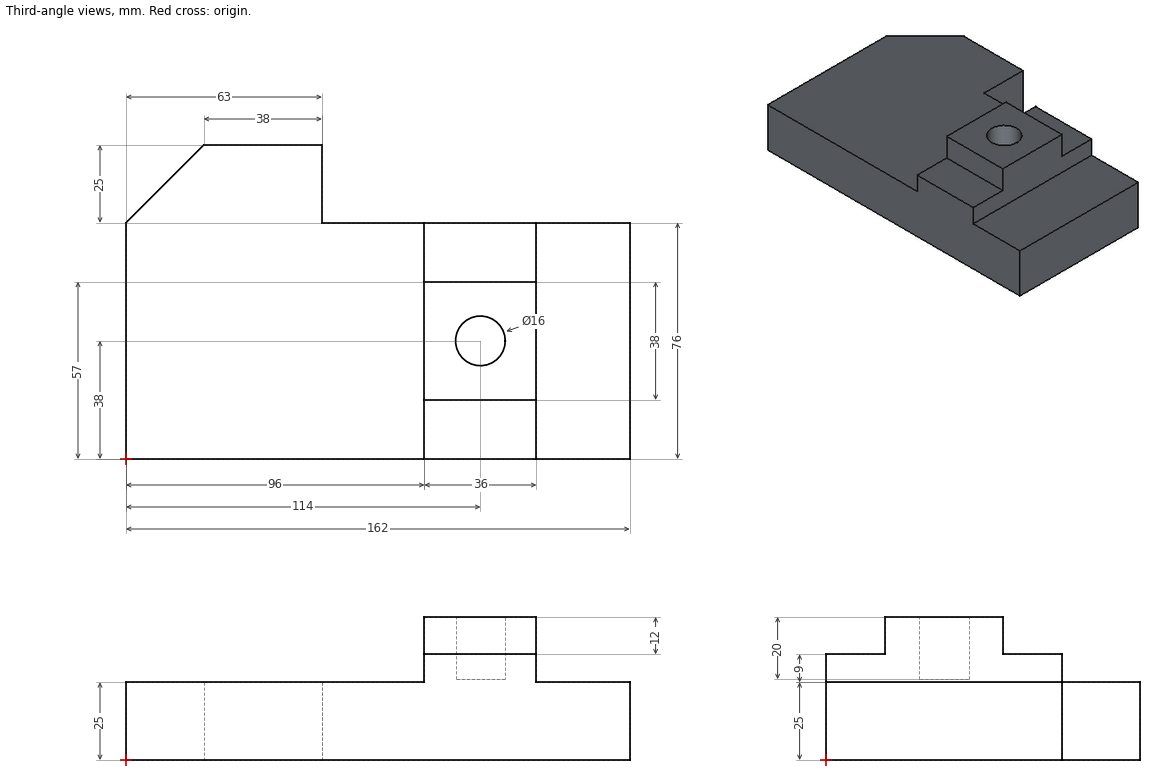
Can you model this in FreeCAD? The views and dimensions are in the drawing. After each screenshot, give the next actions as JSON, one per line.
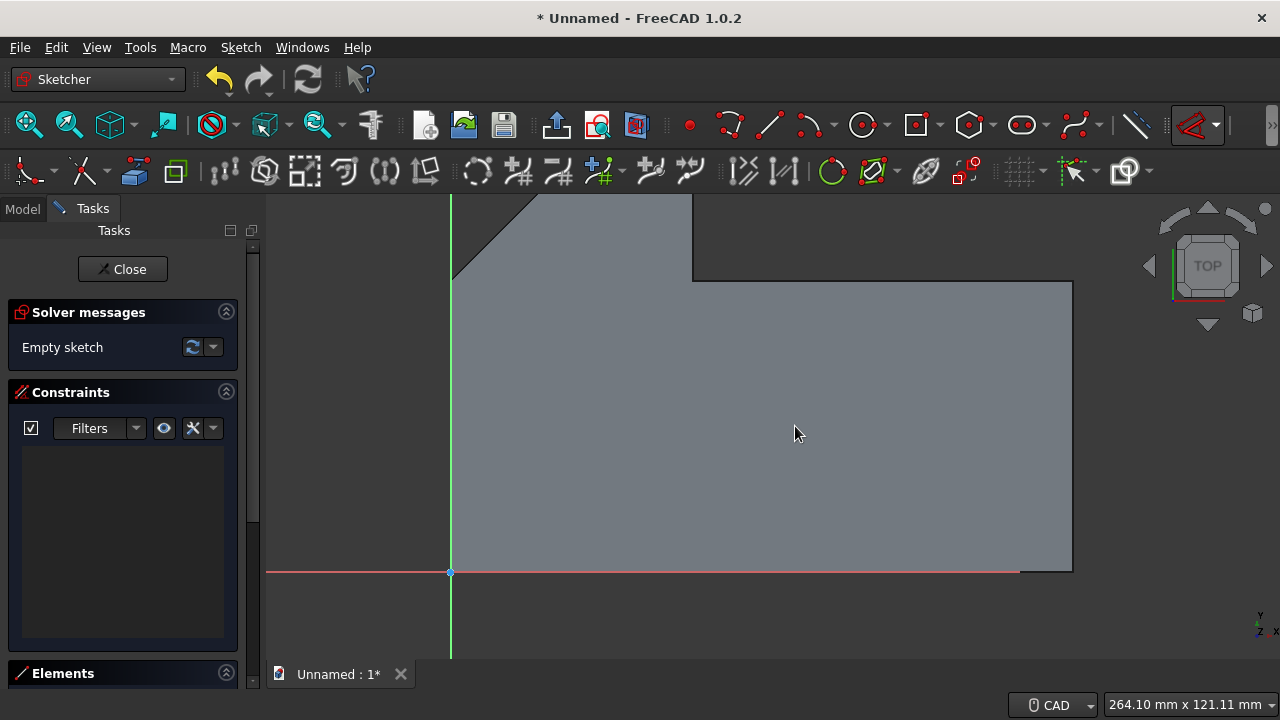
{"action": "key", "text": "g r"}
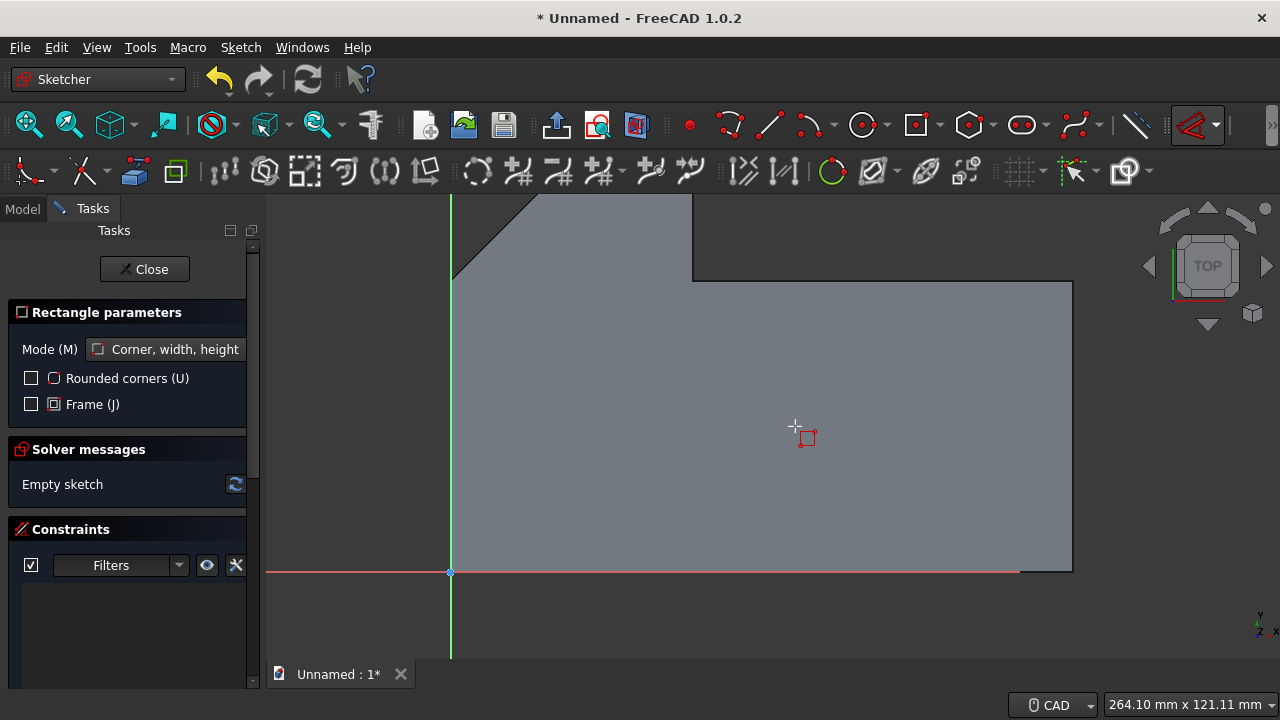
{"action": "left_click", "coordinate": [820, 281]}
{"action": "left_click", "coordinate": [958, 572]}
{"action": "key", "text": "Escape"}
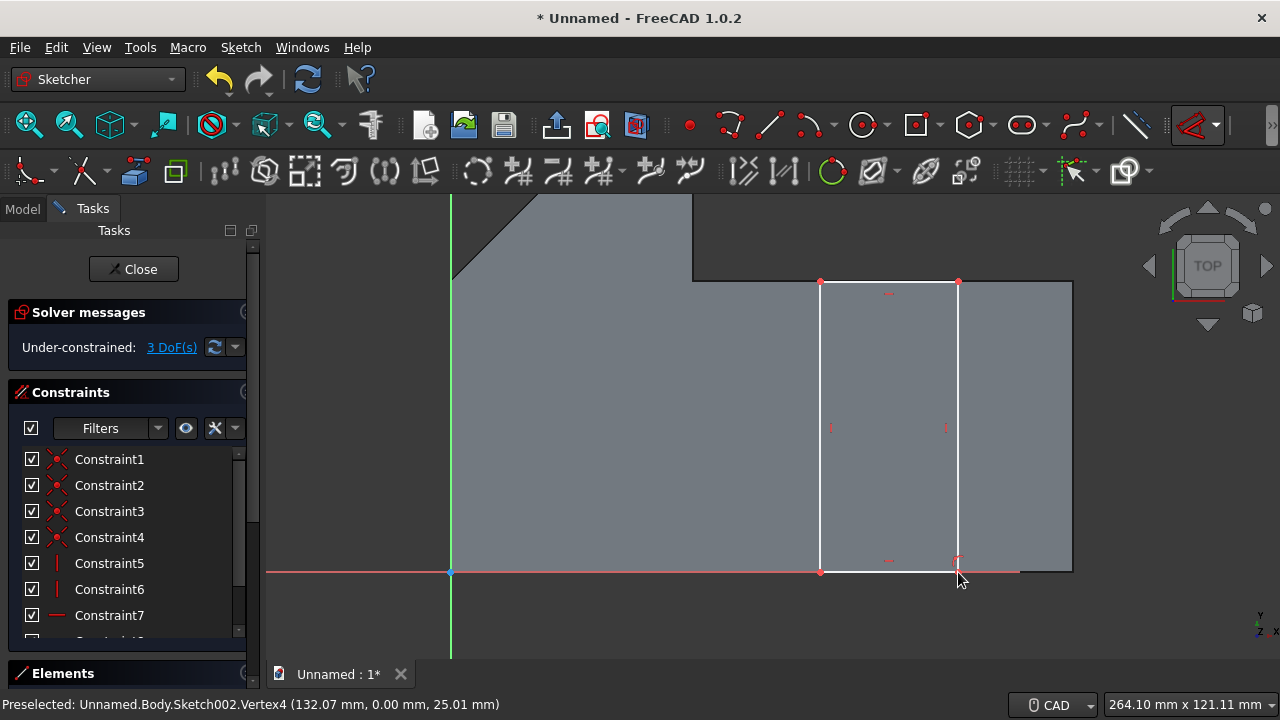
{"action": "left_click", "coordinate": [820, 369]}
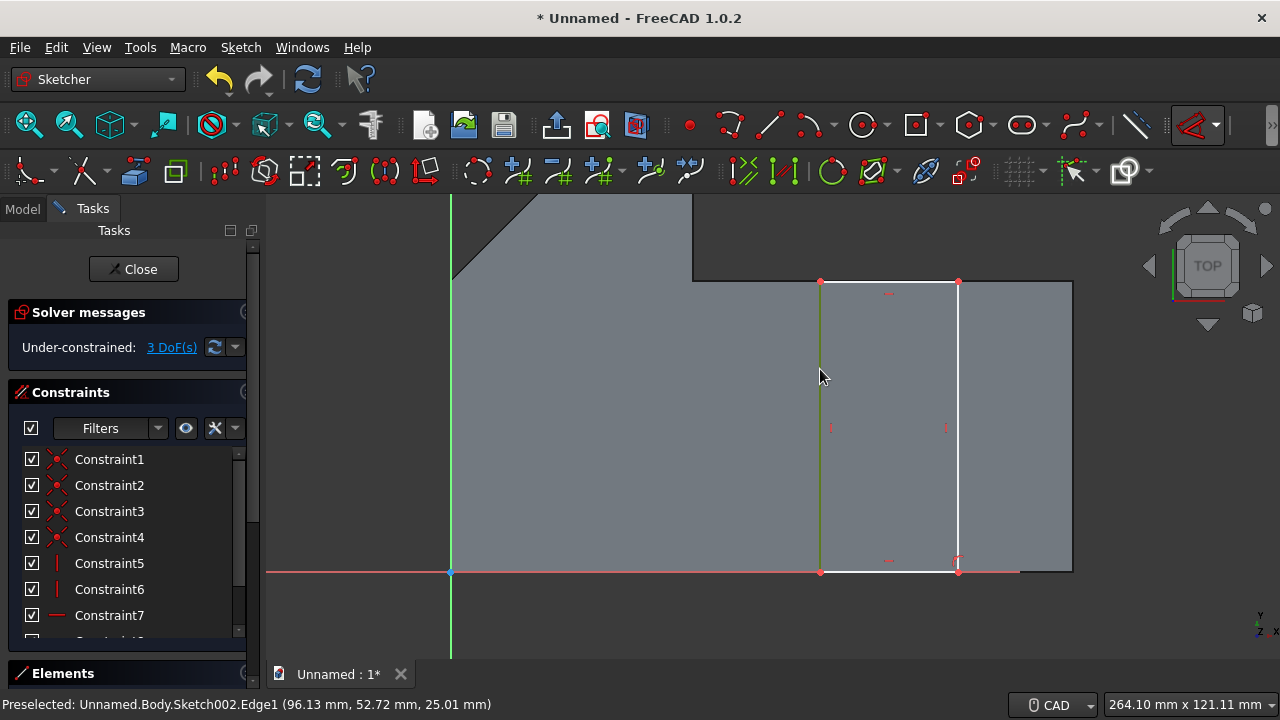
{"action": "left_click", "coordinate": [1218, 126]}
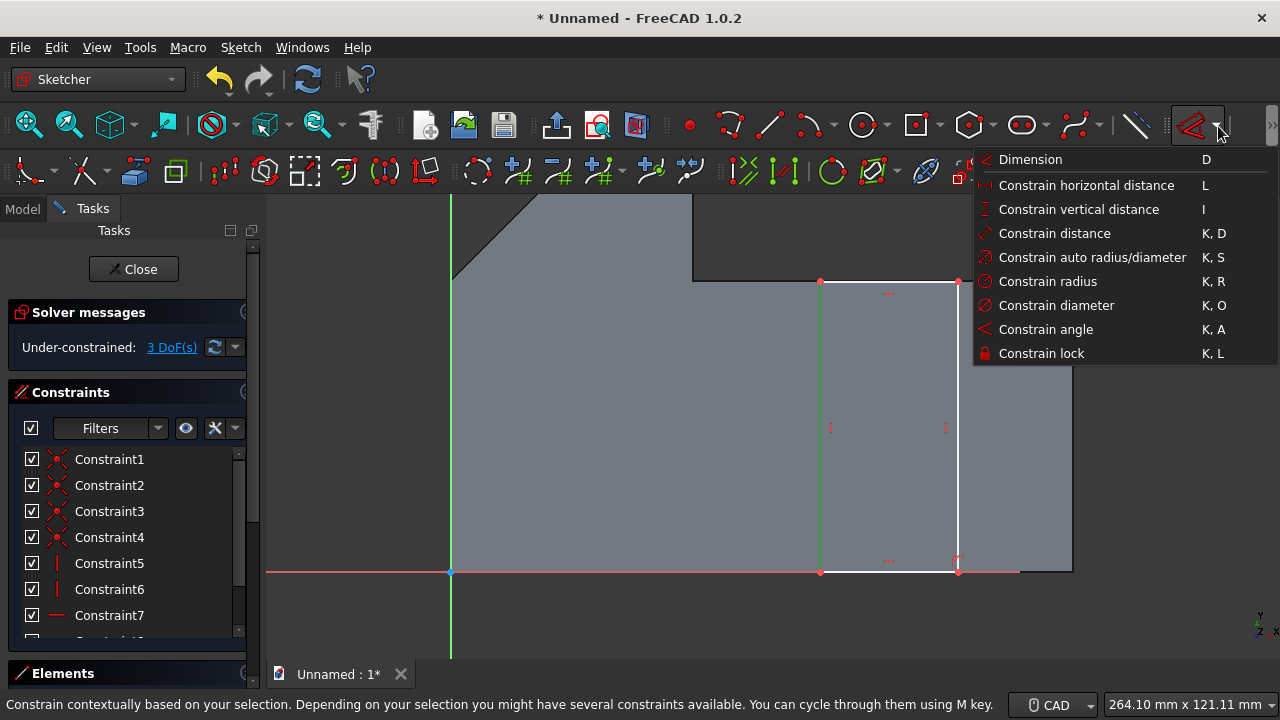
{"action": "left_click", "coordinate": [1126, 209]}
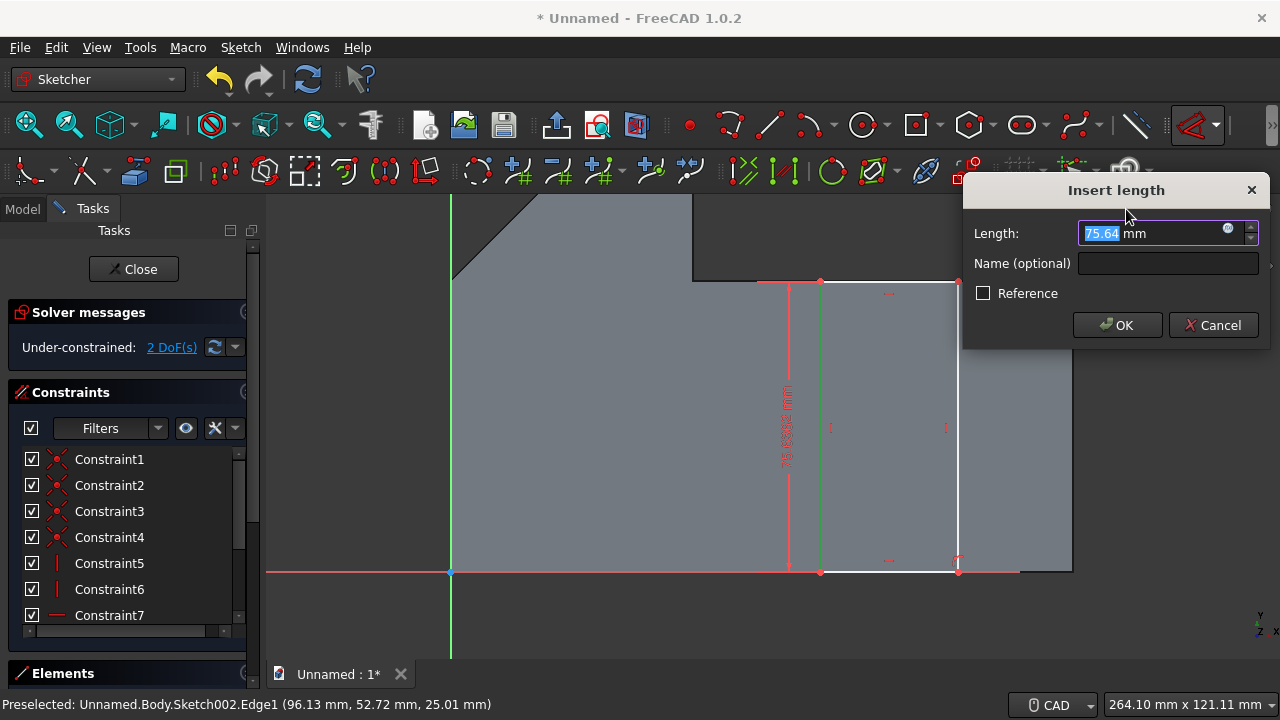
{"action": "type", "text": "76"}
{"action": "key", "text": "Return"}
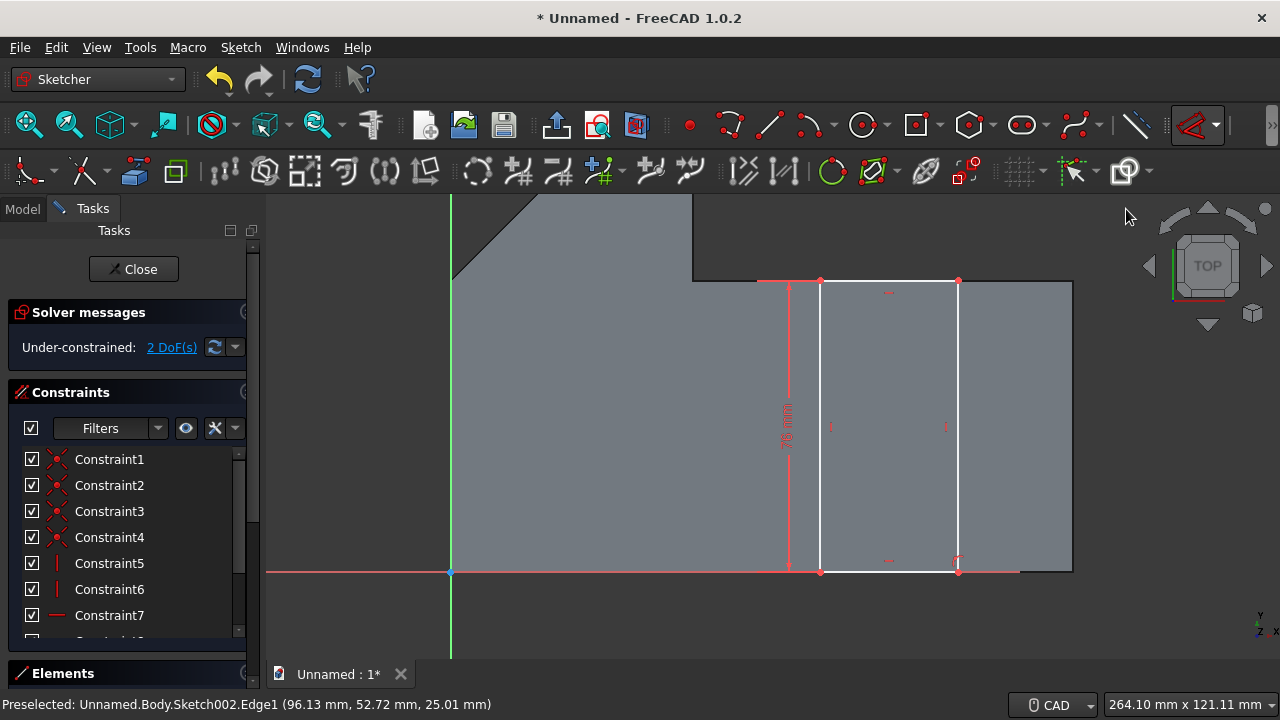
{"action": "left_click", "coordinate": [861, 572]}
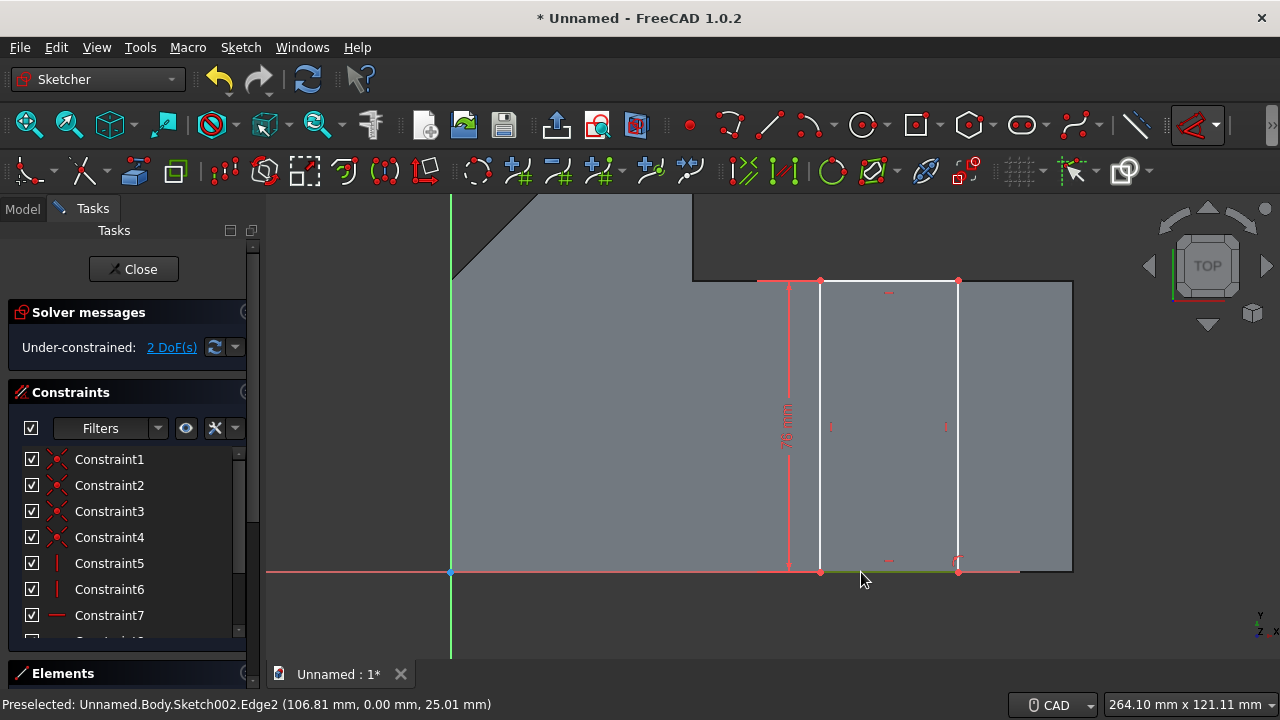
{"action": "key", "text": "l"}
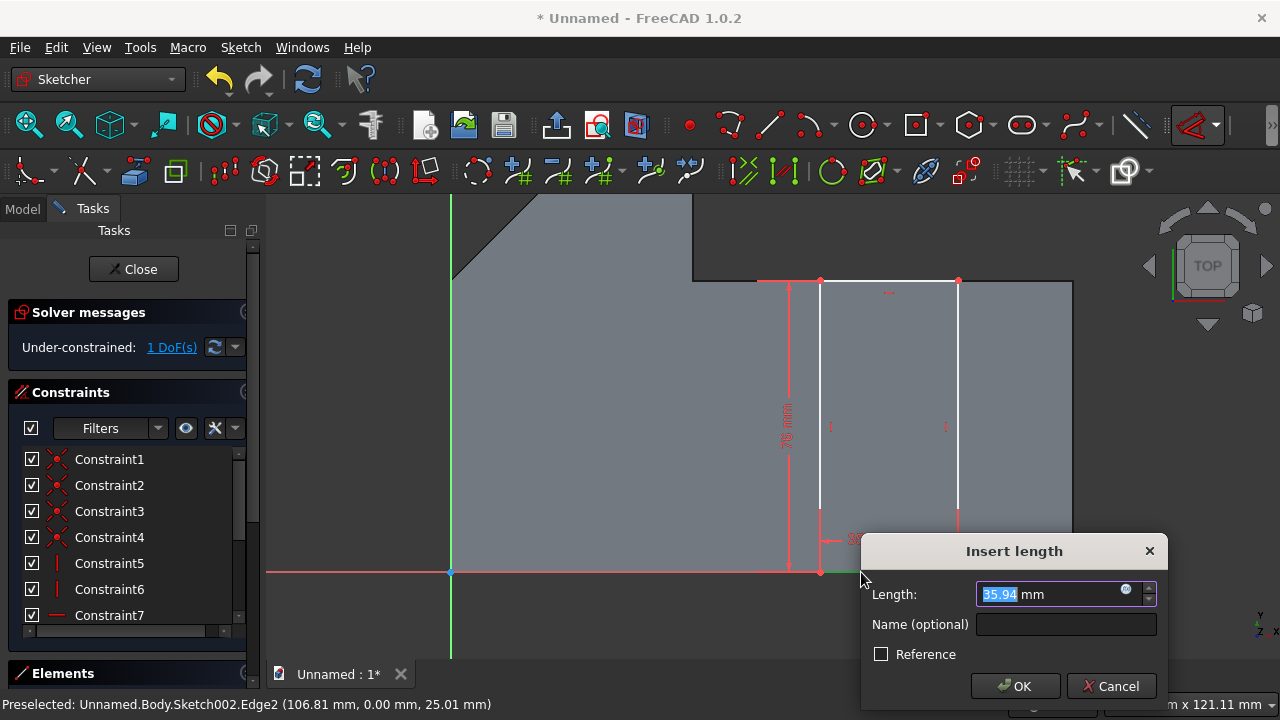
{"action": "type", "text": "36"}
{"action": "key", "text": "Return"}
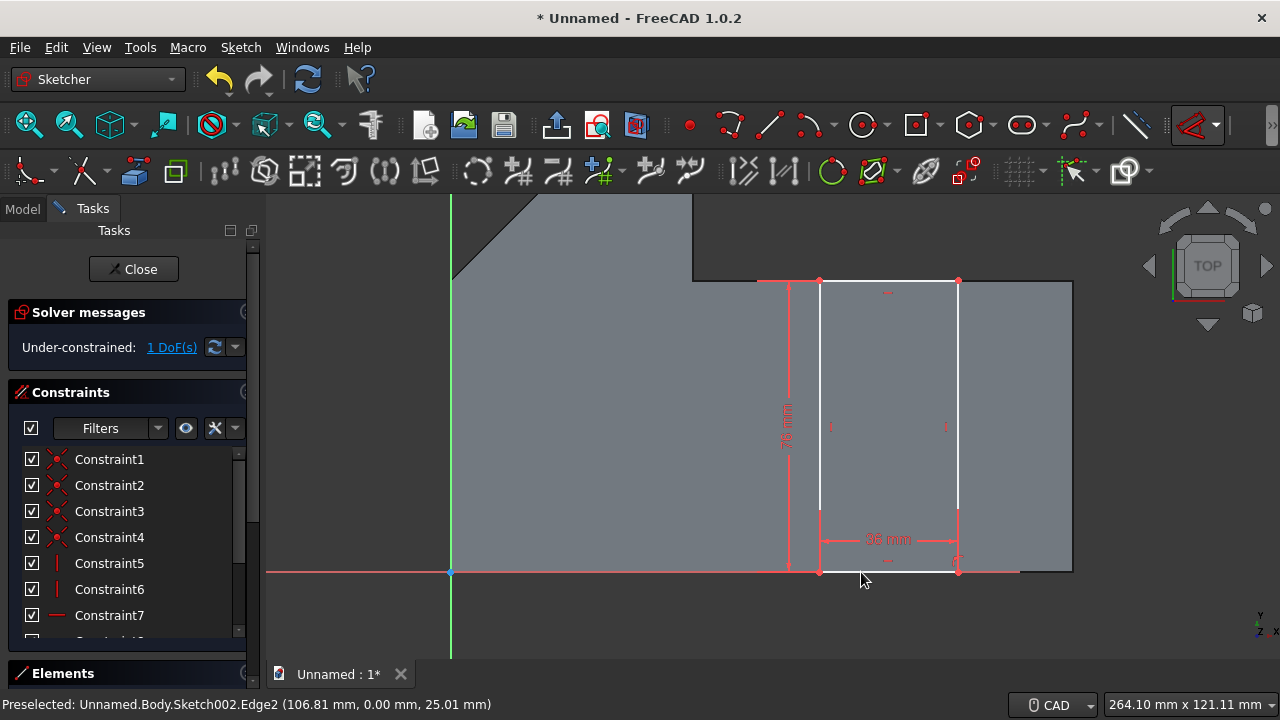
{"action": "left_click", "coordinate": [820, 281]}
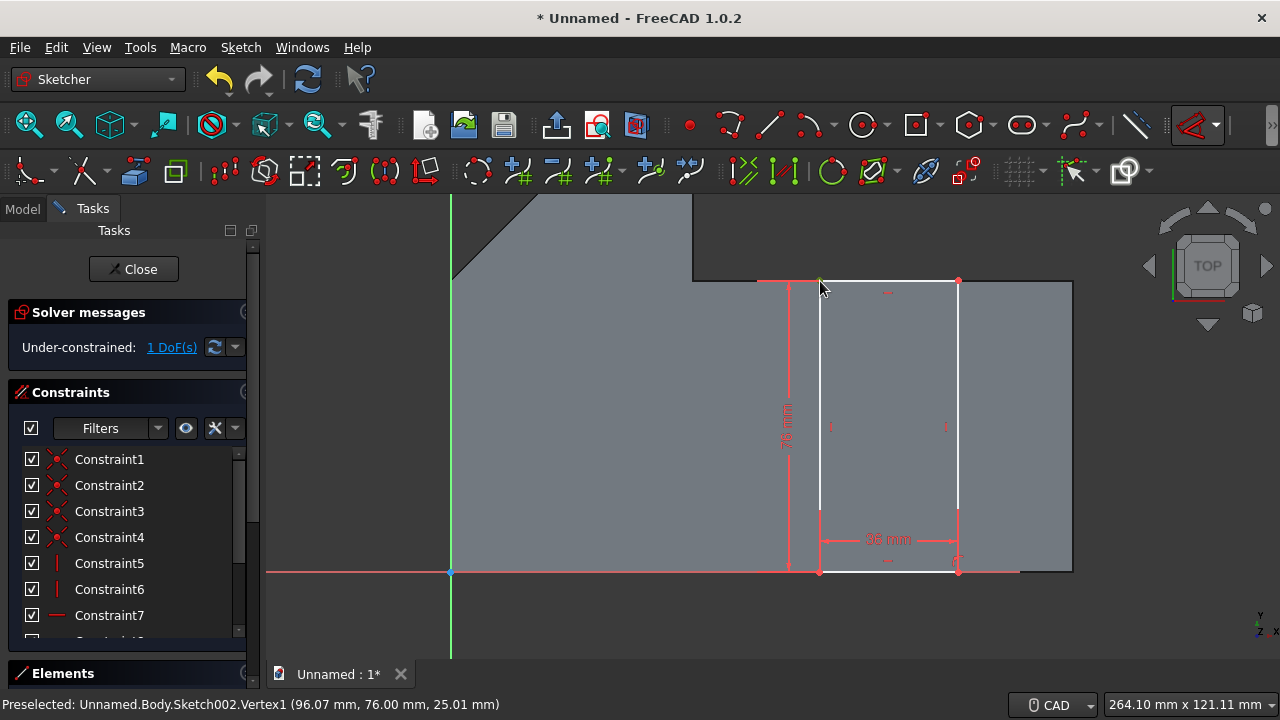
{"action": "left_click", "coordinate": [1218, 126]}